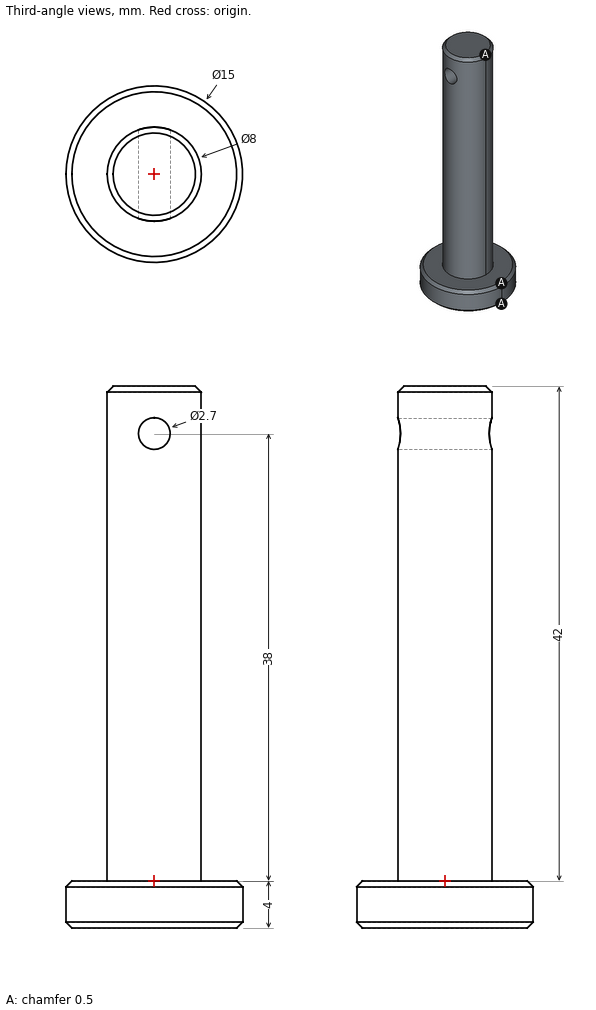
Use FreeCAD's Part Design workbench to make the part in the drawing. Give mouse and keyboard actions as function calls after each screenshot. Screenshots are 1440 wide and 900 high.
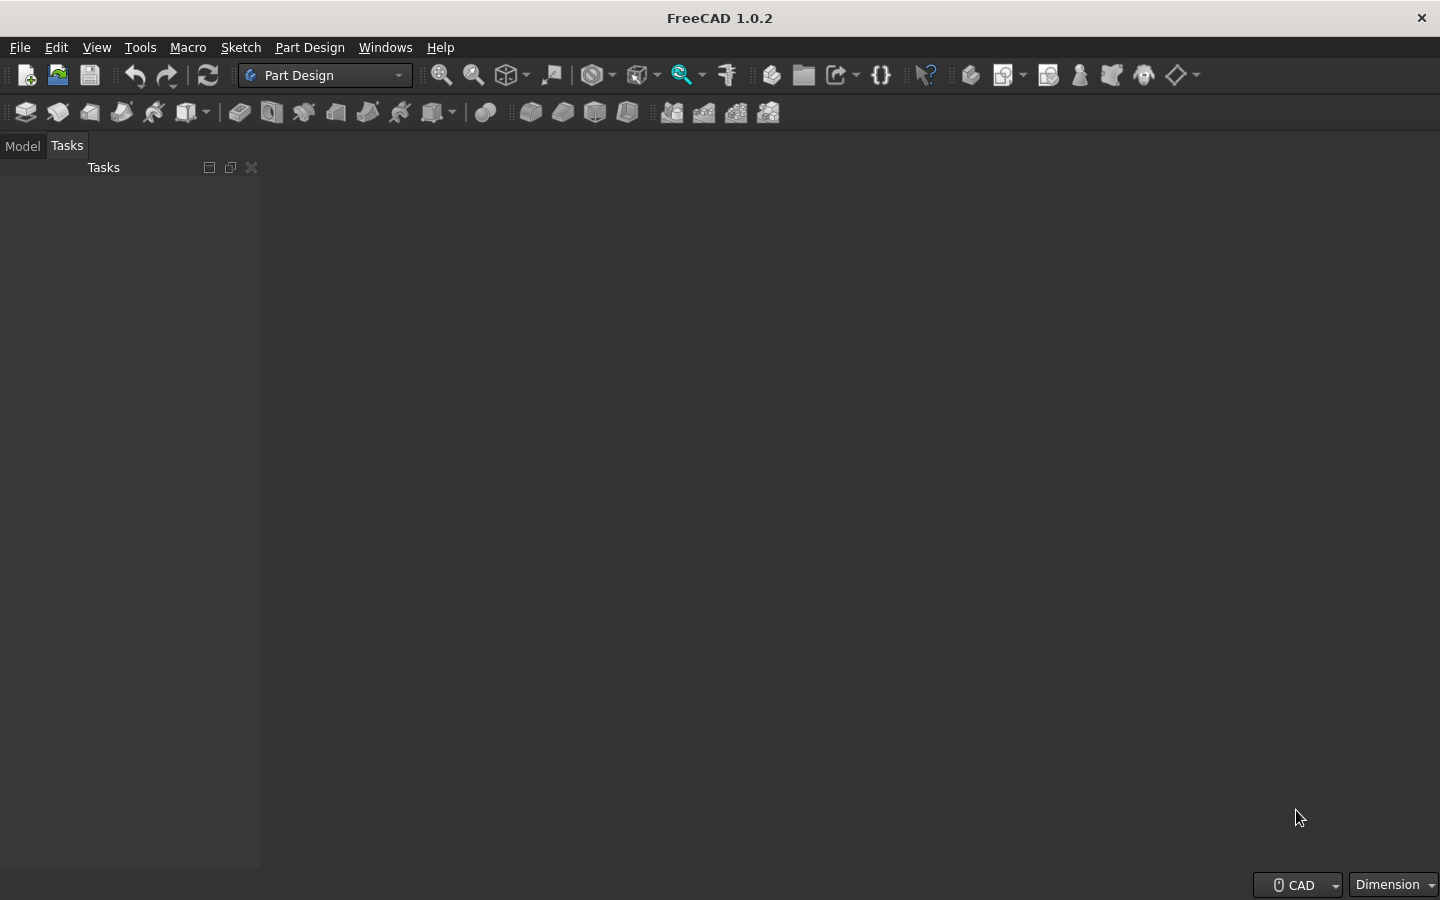
key(ctrl+n)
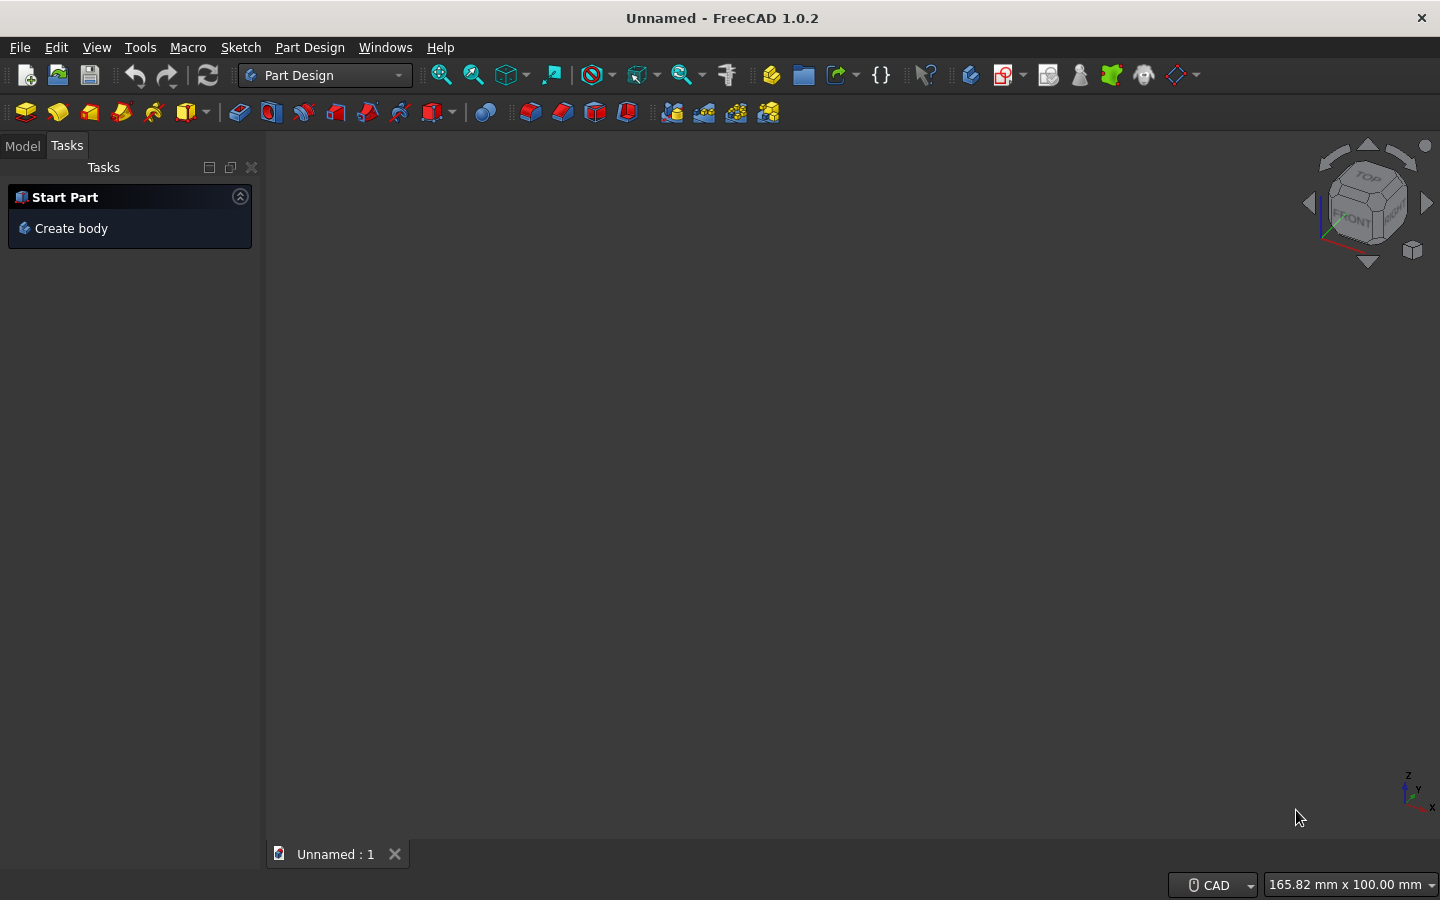
click(1004, 76)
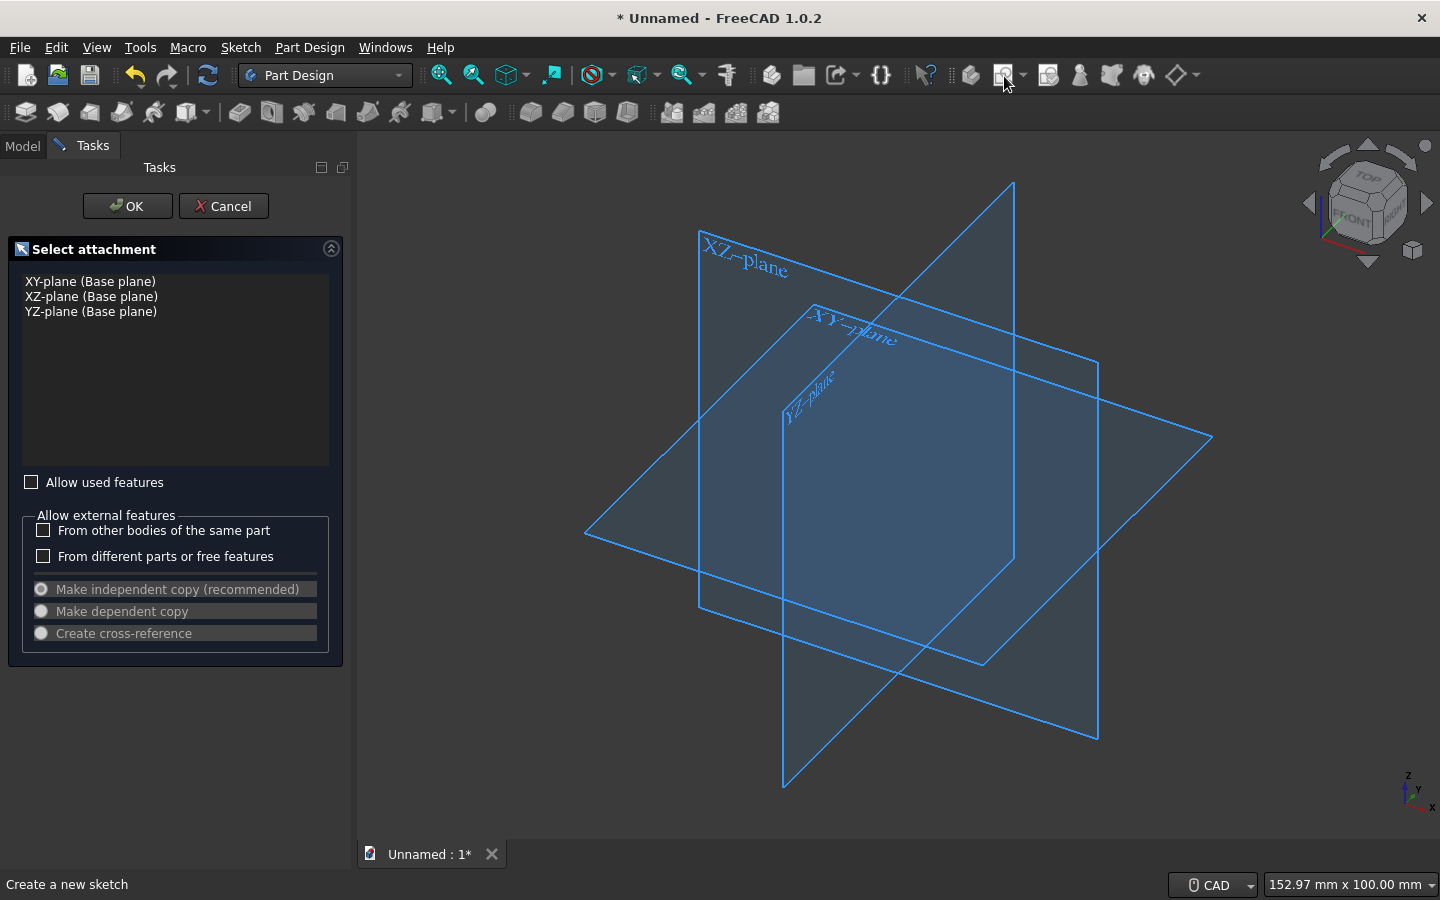
click(82, 282)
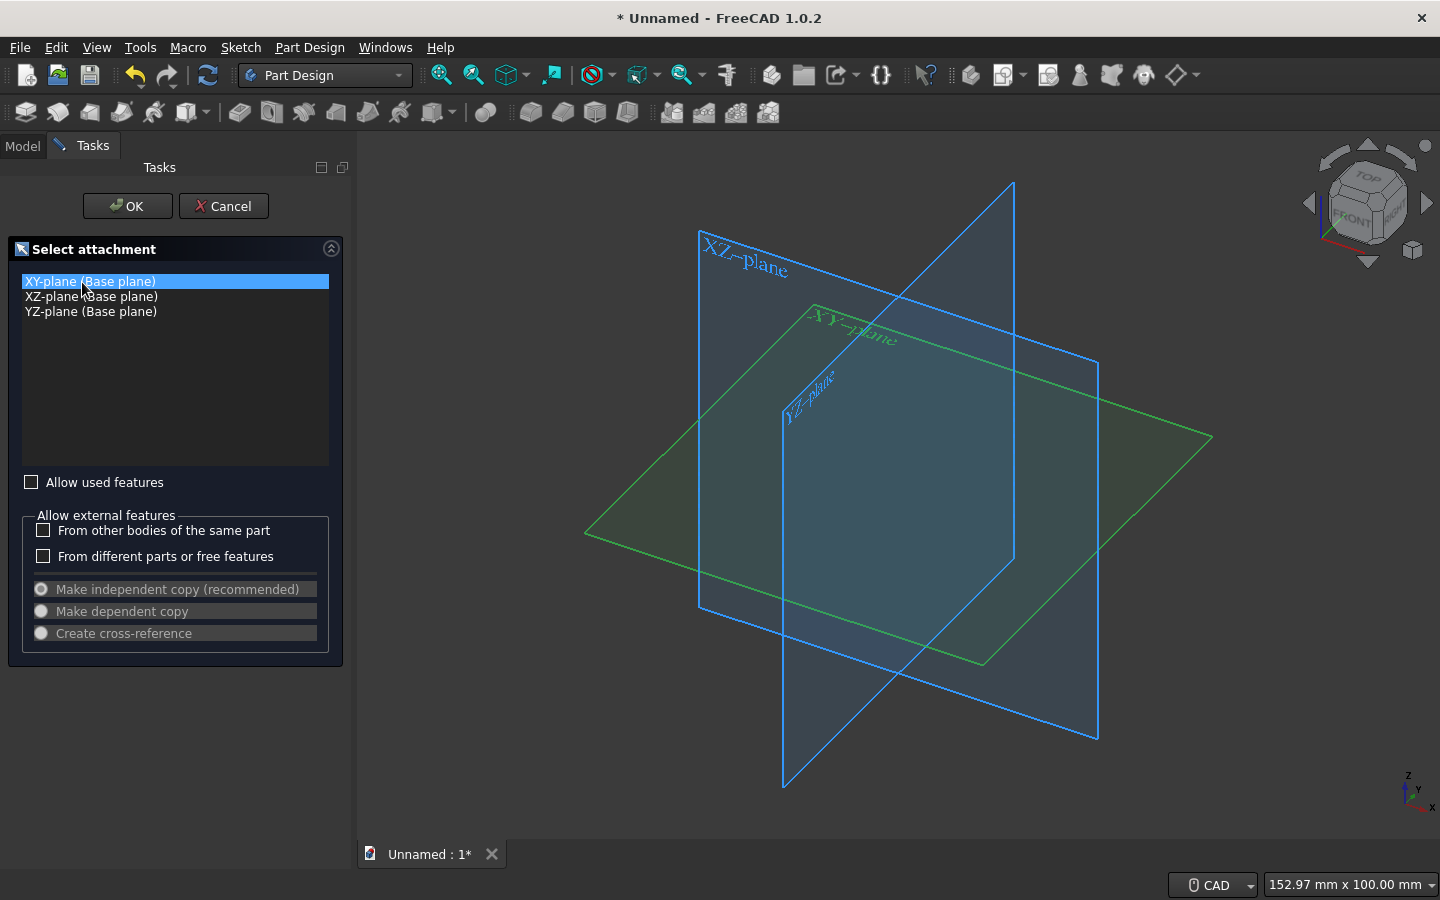
click(128, 206)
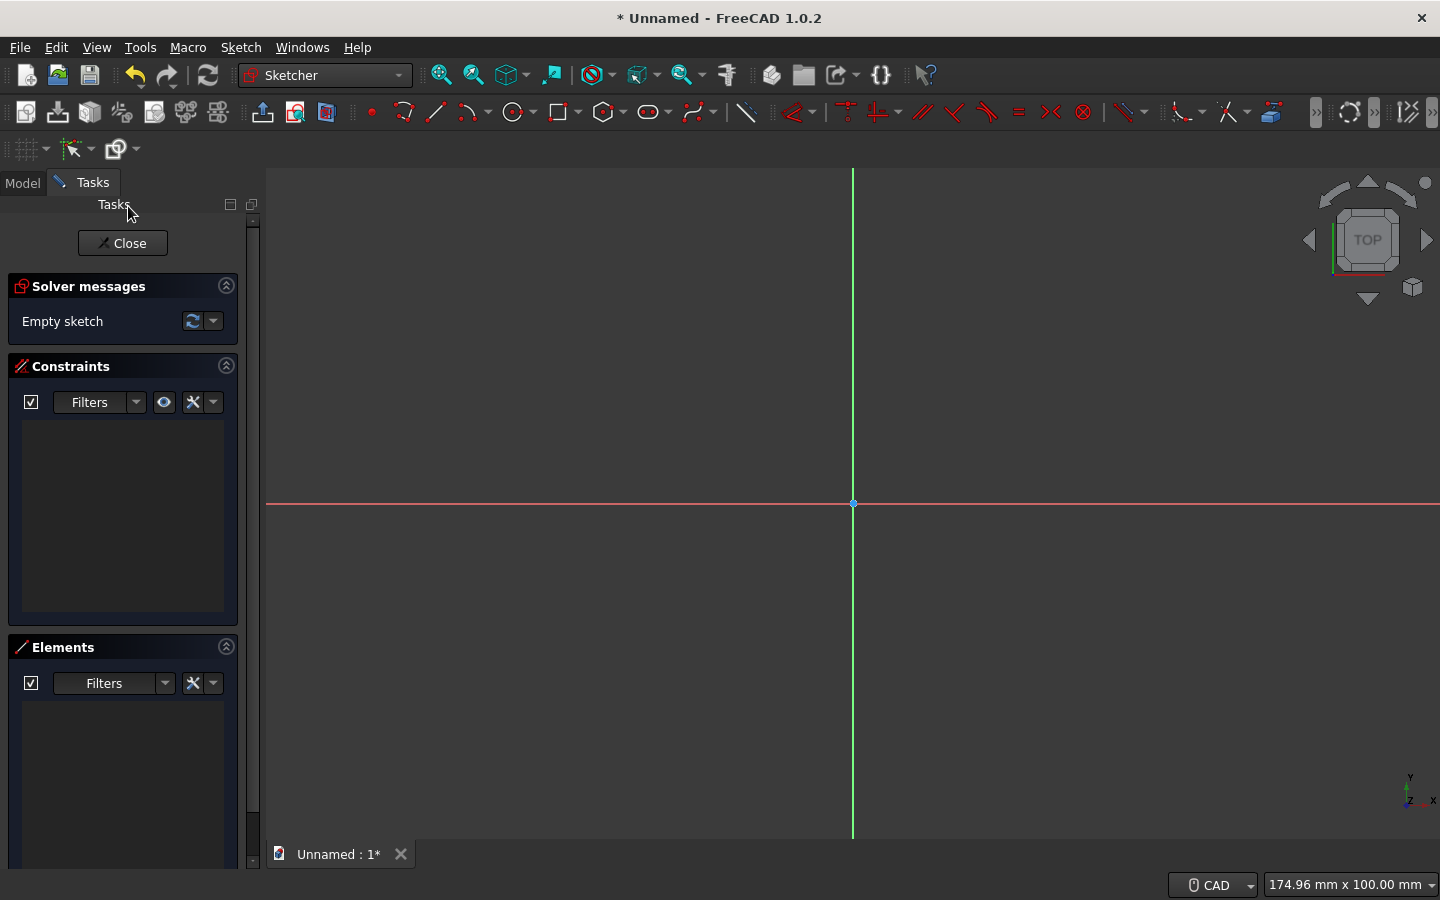
scroll(864, 504, up, 10)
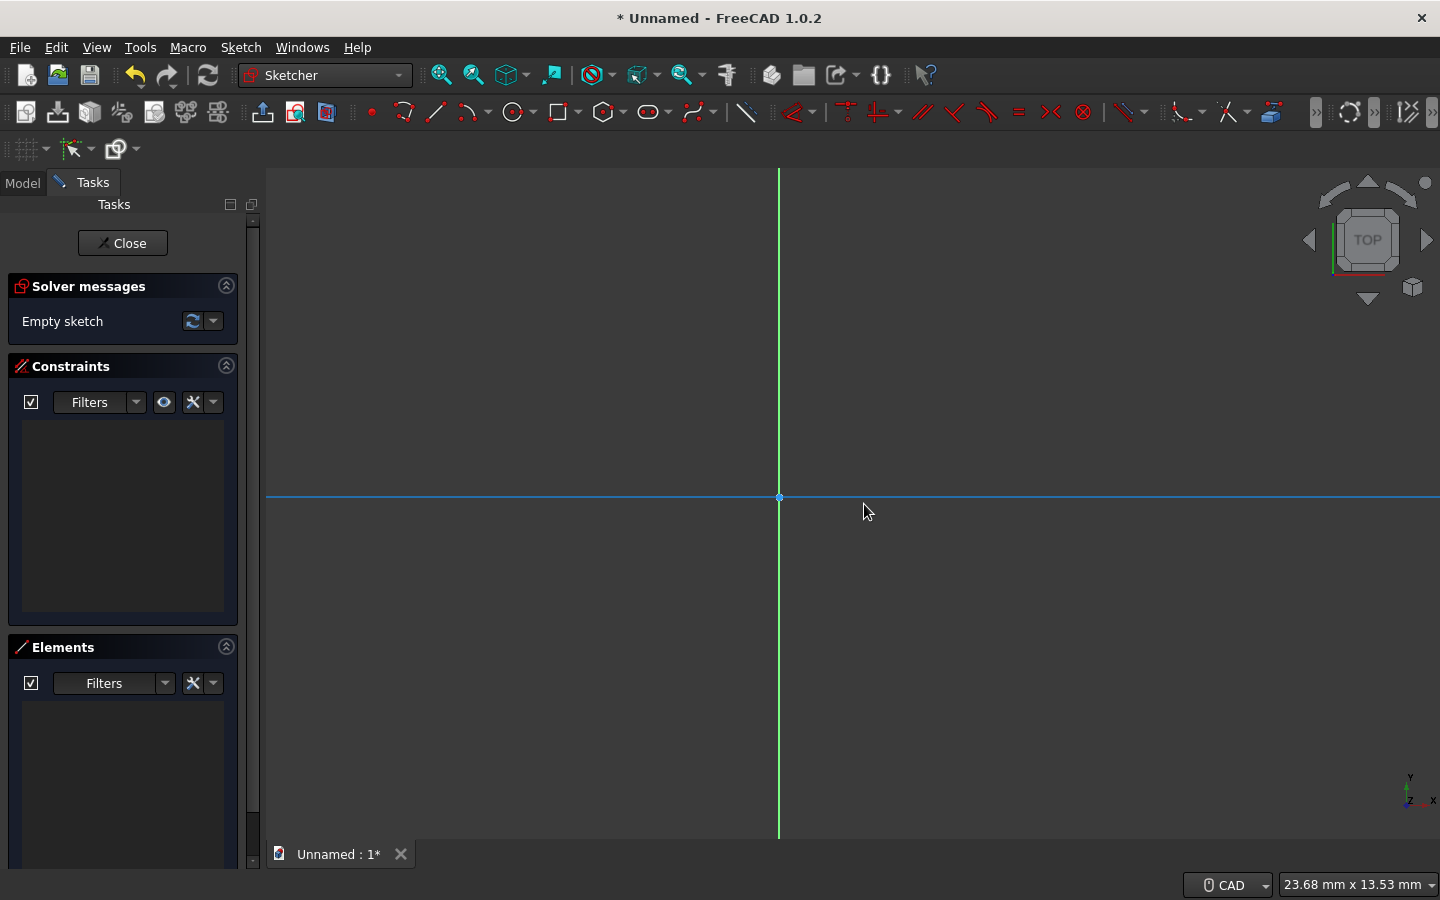
key(g)
key(c)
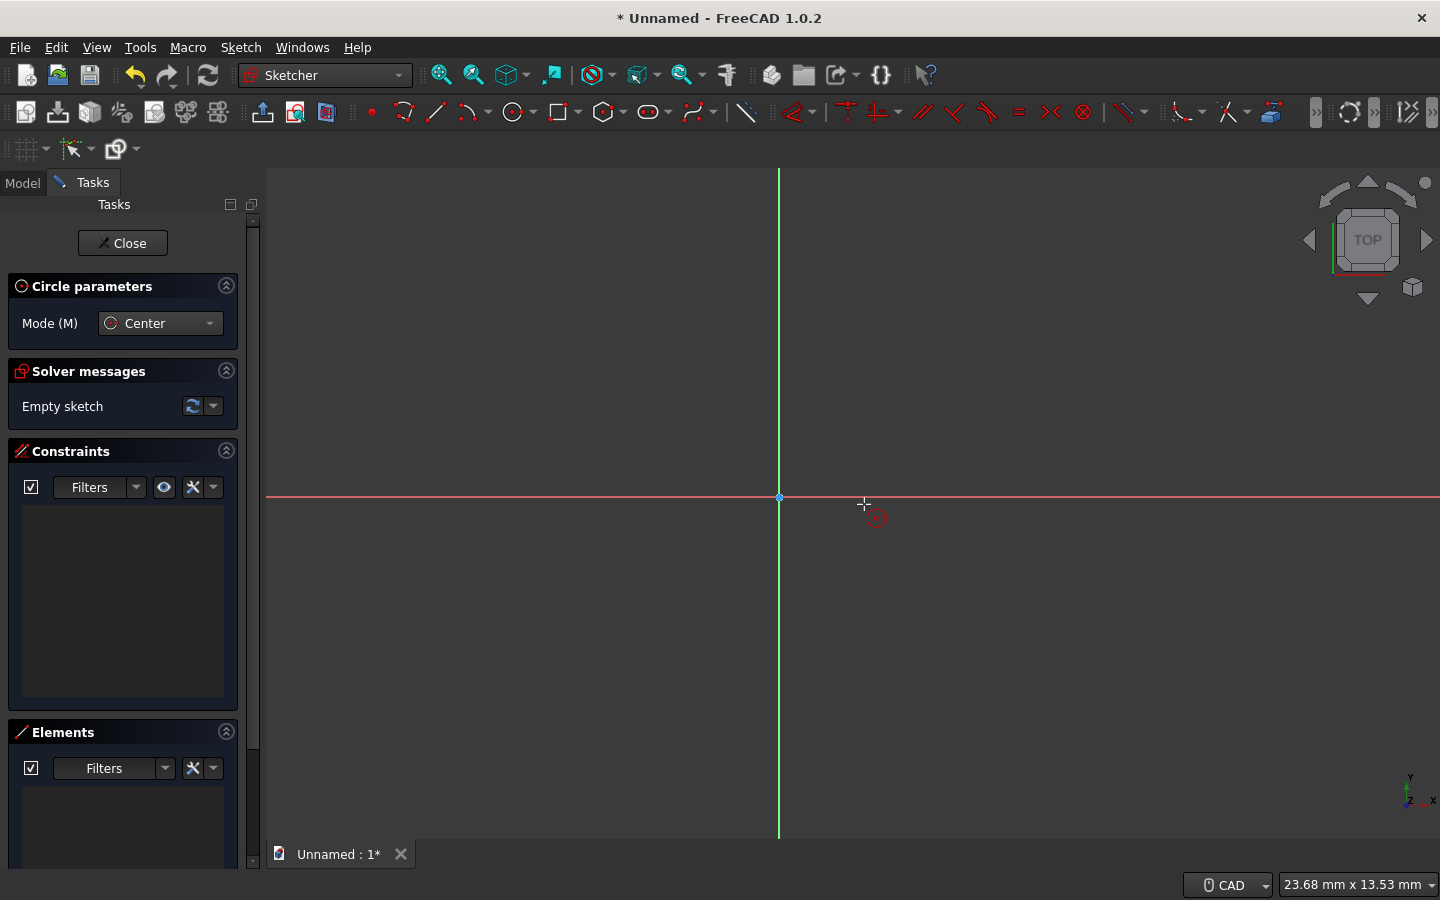
click(779, 497)
move(920, 357)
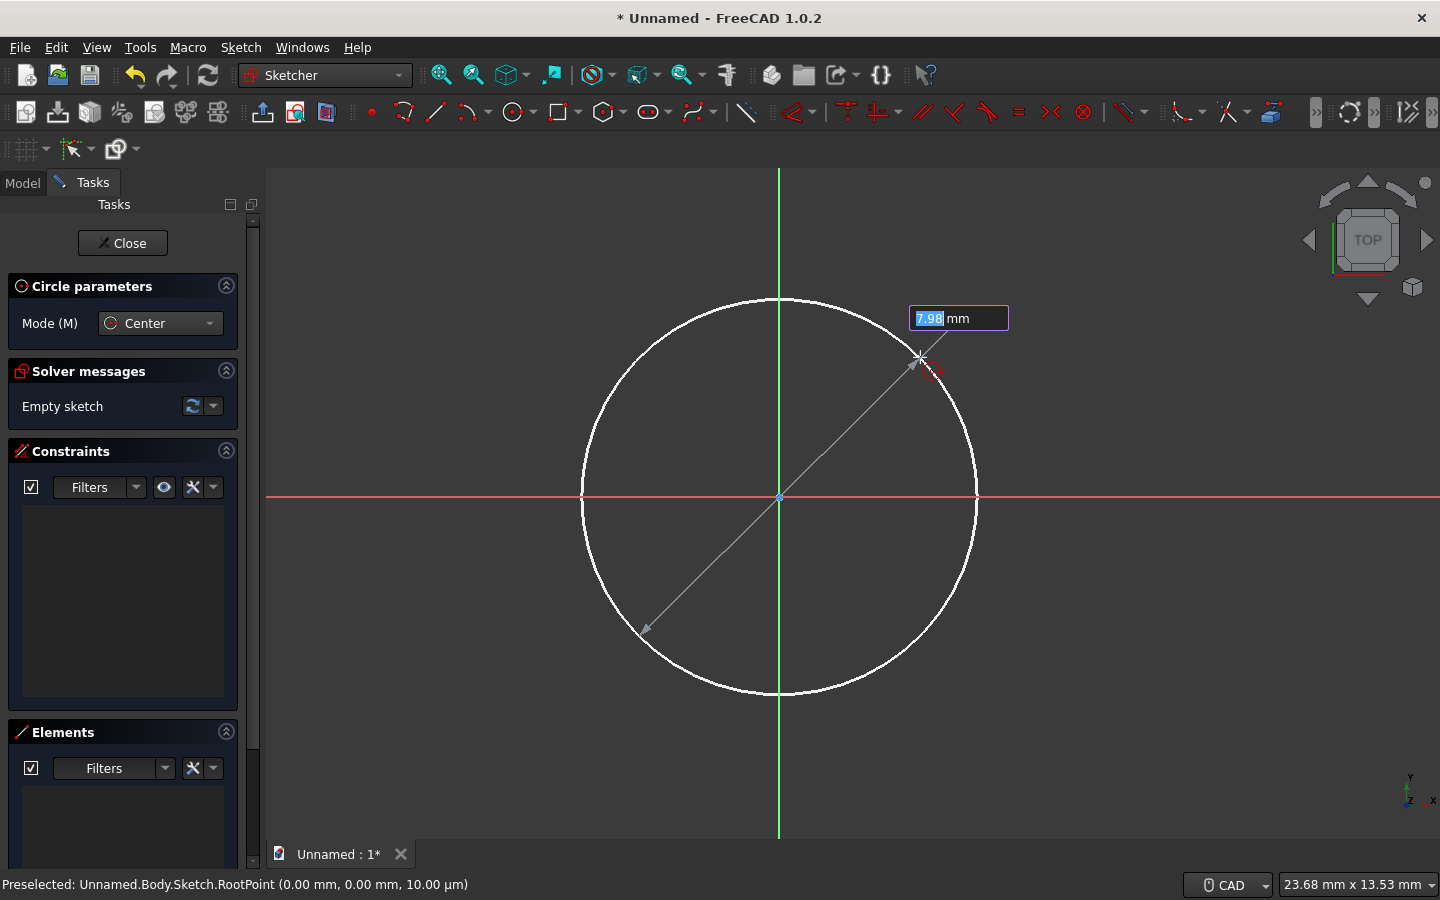
text(8)
key(Return)
key(Escape)